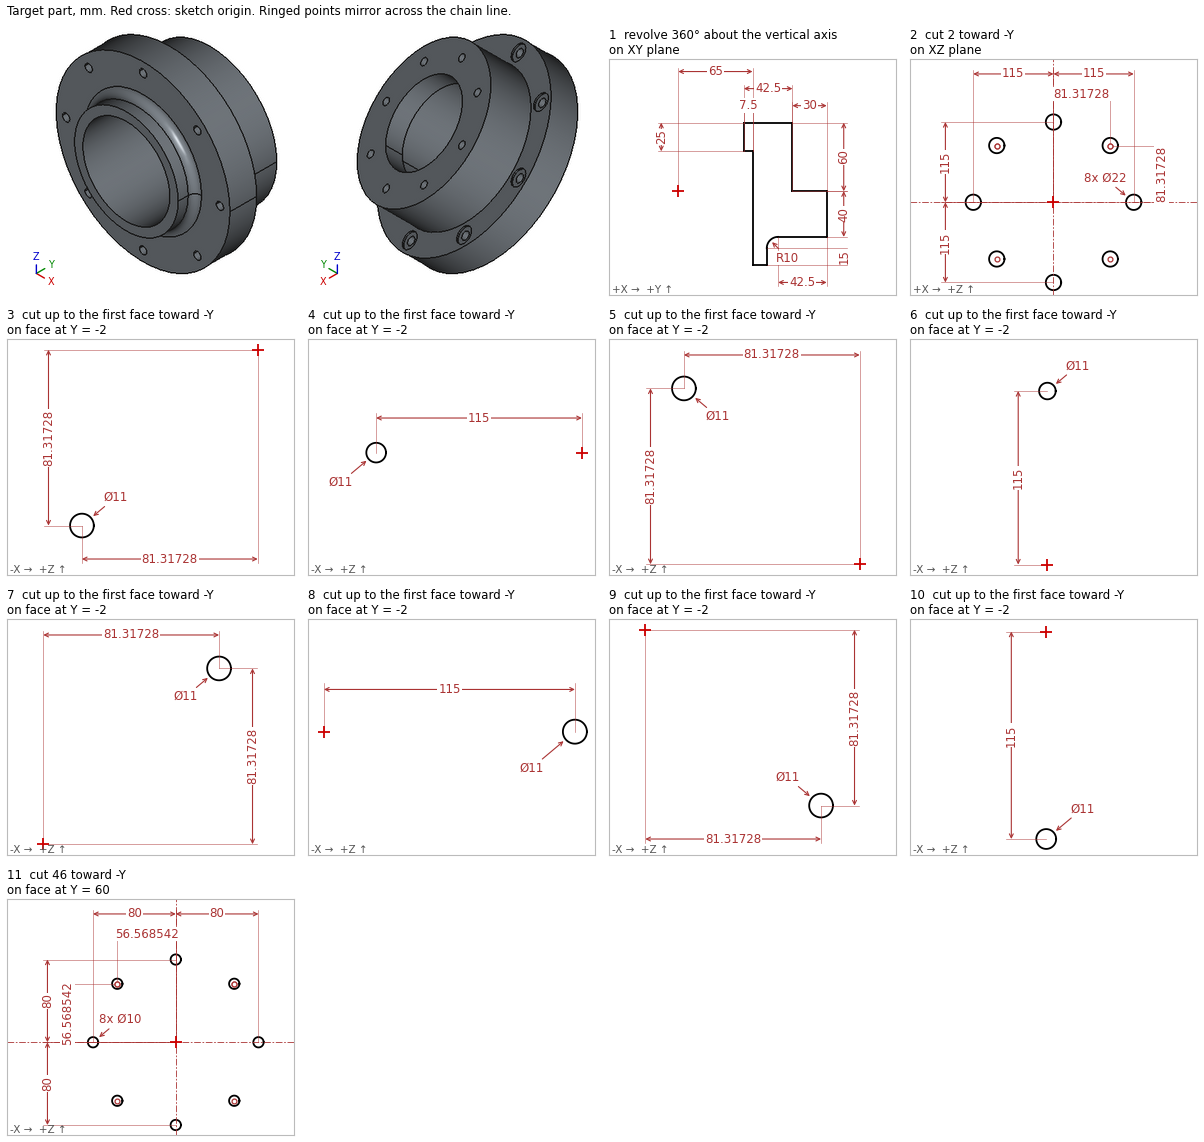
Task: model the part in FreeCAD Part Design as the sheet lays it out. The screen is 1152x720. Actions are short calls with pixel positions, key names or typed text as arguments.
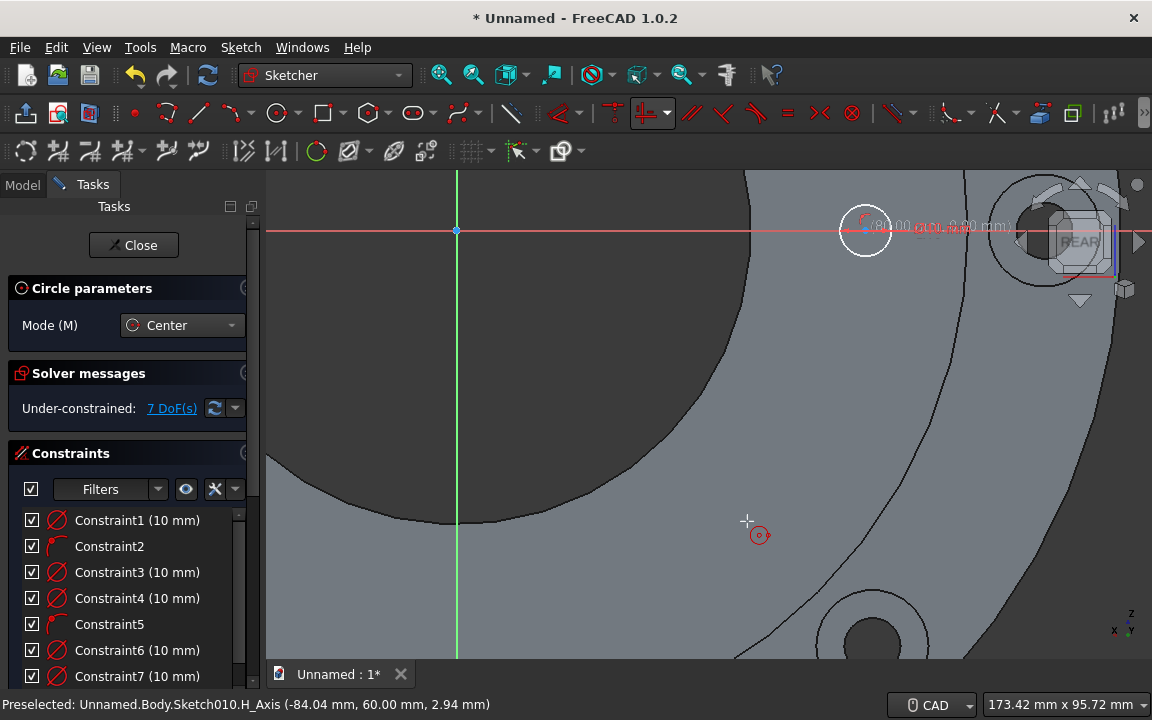
click(746, 520)
move(764, 502)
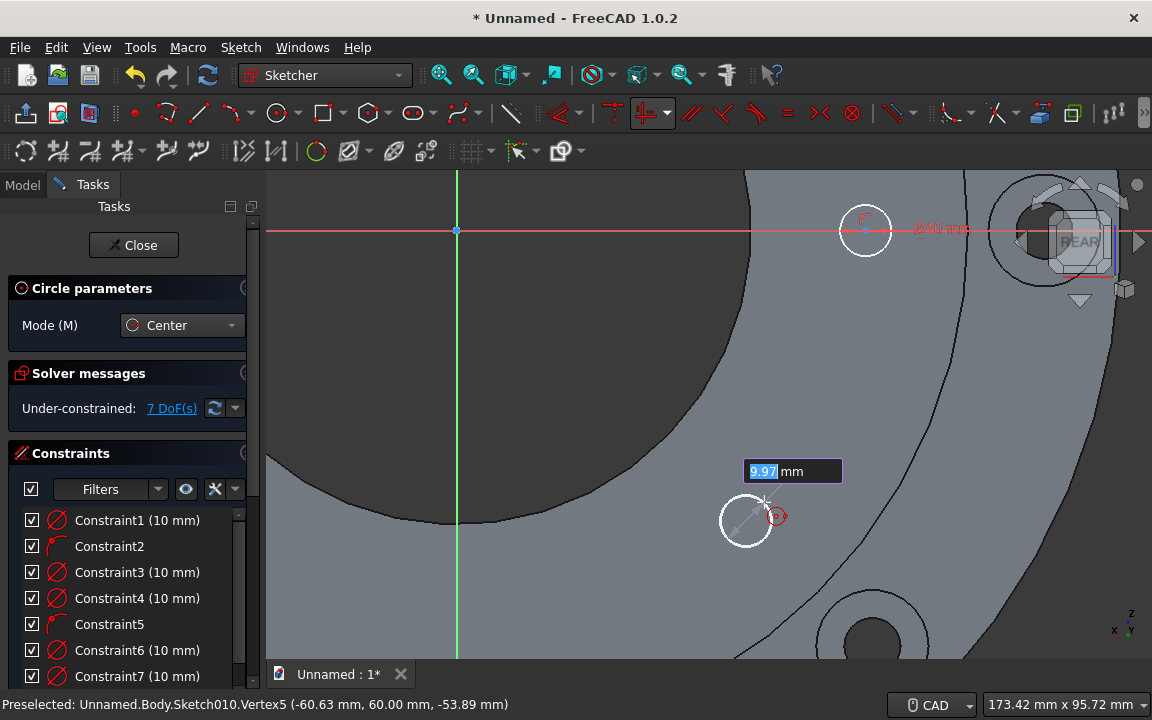
text(10)
key(Return)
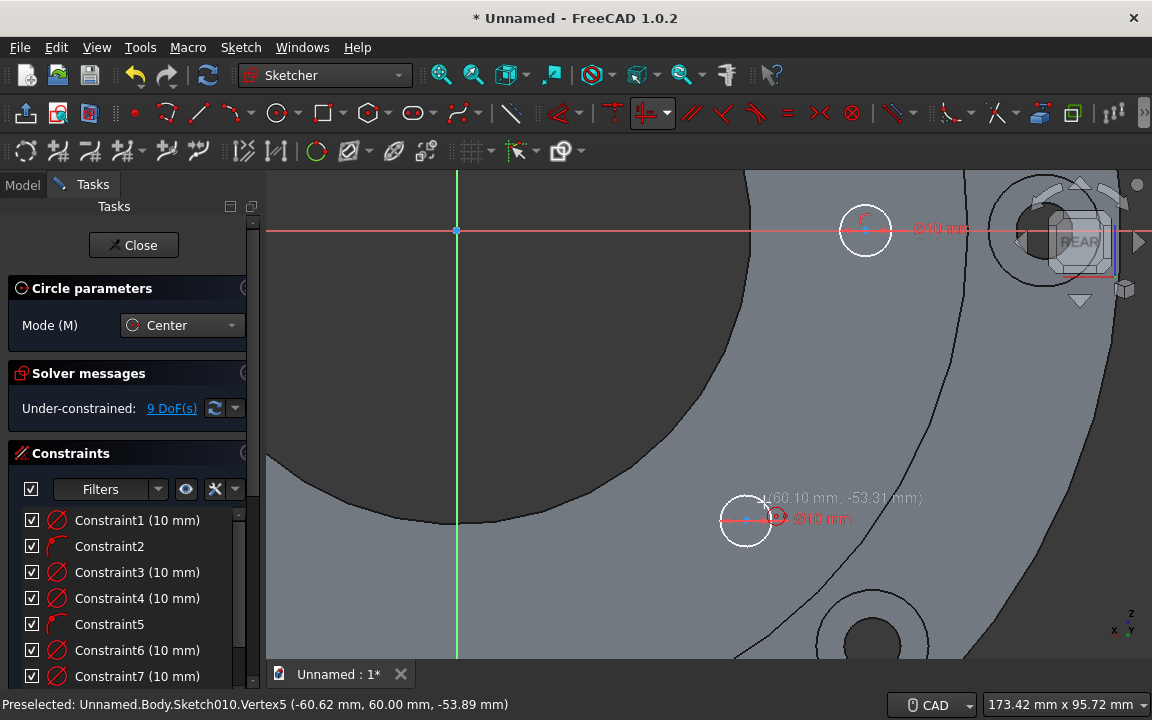
scroll(747, 521, down, 5)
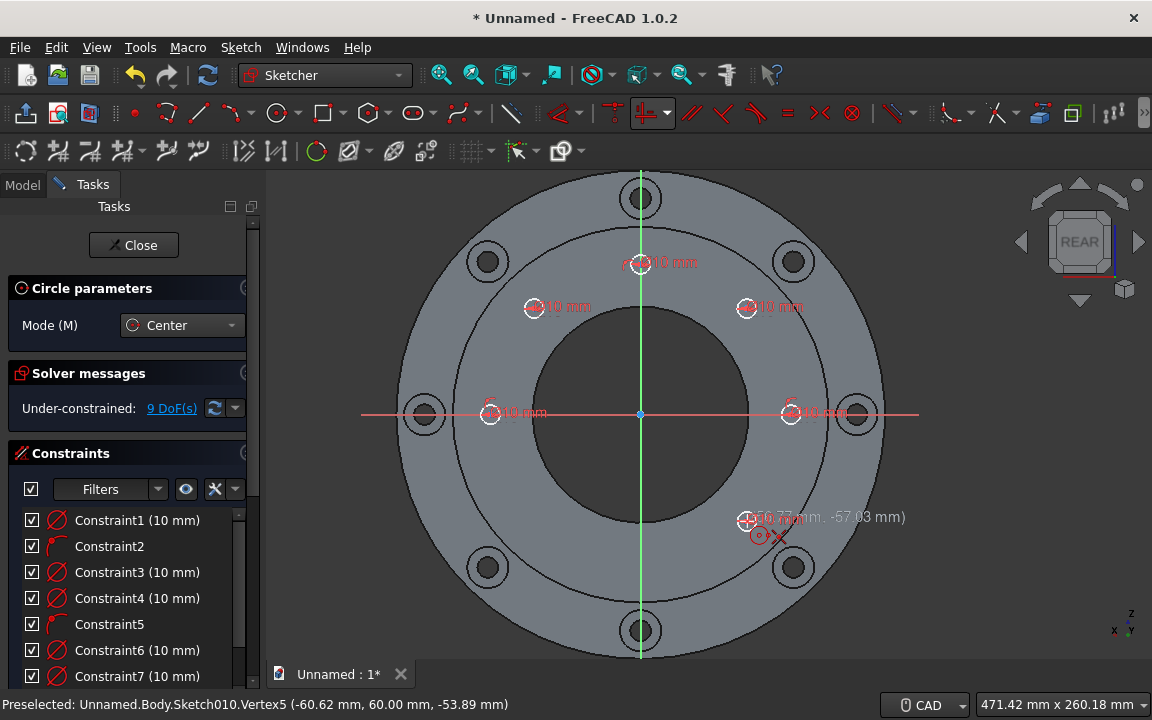
scroll(641, 565, up, 5)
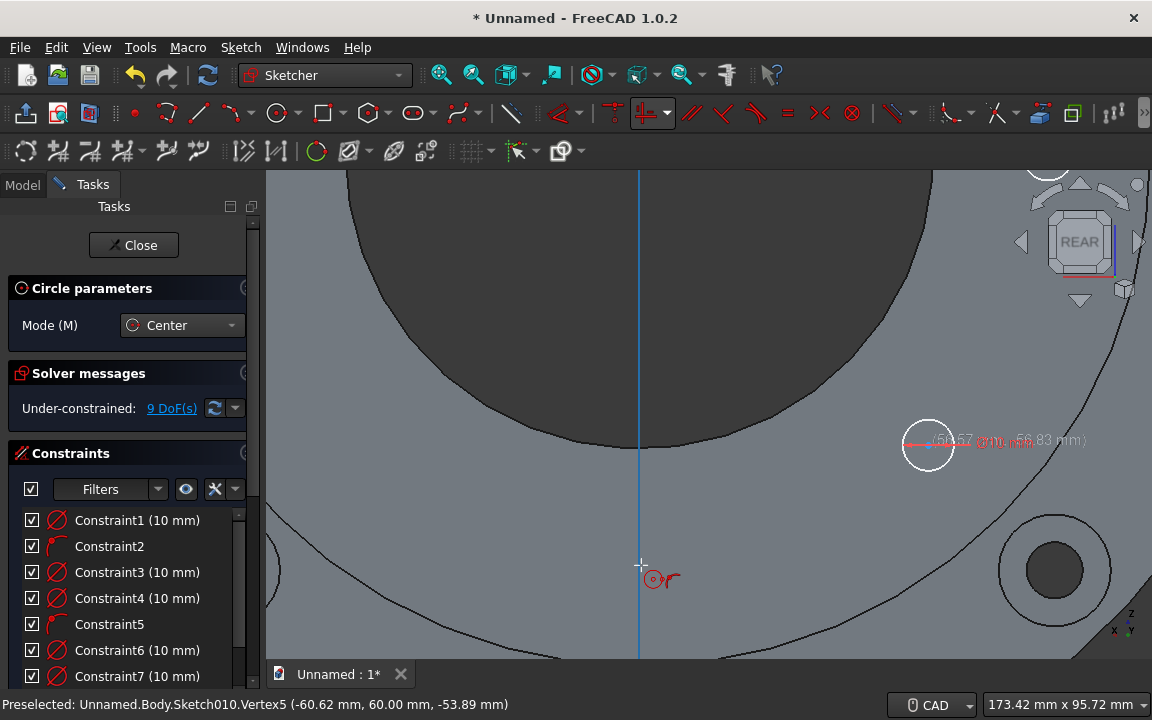
click(639, 564)
move(657, 546)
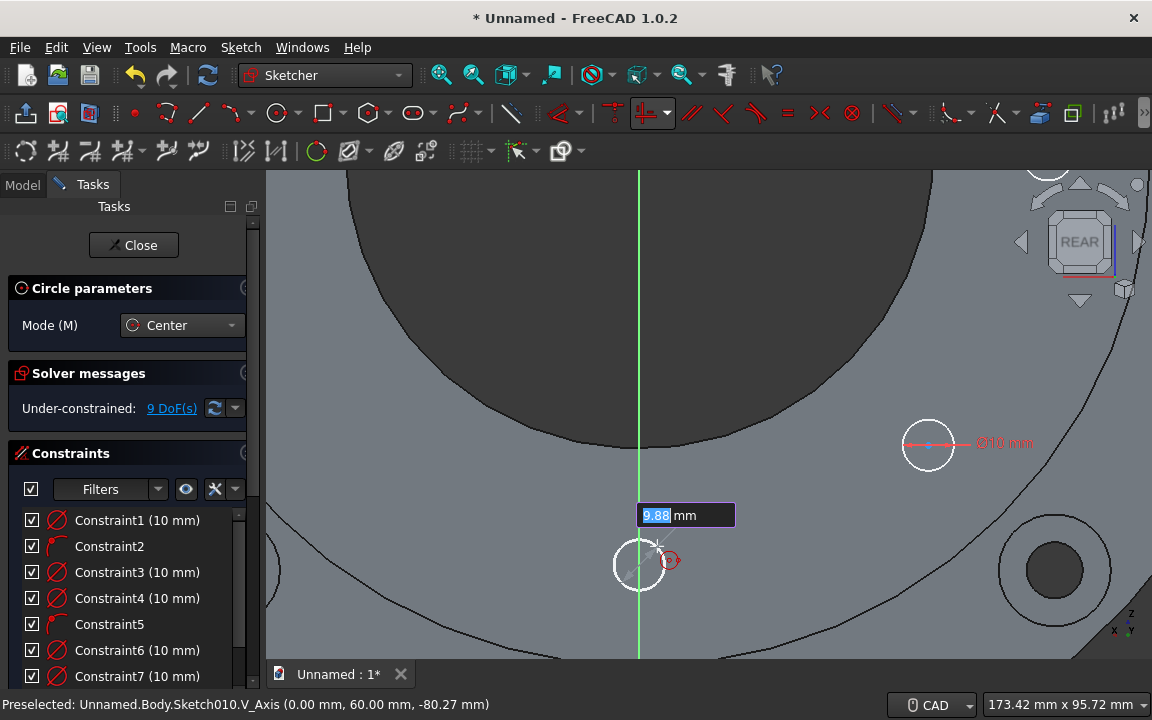
text(10)
key(Return)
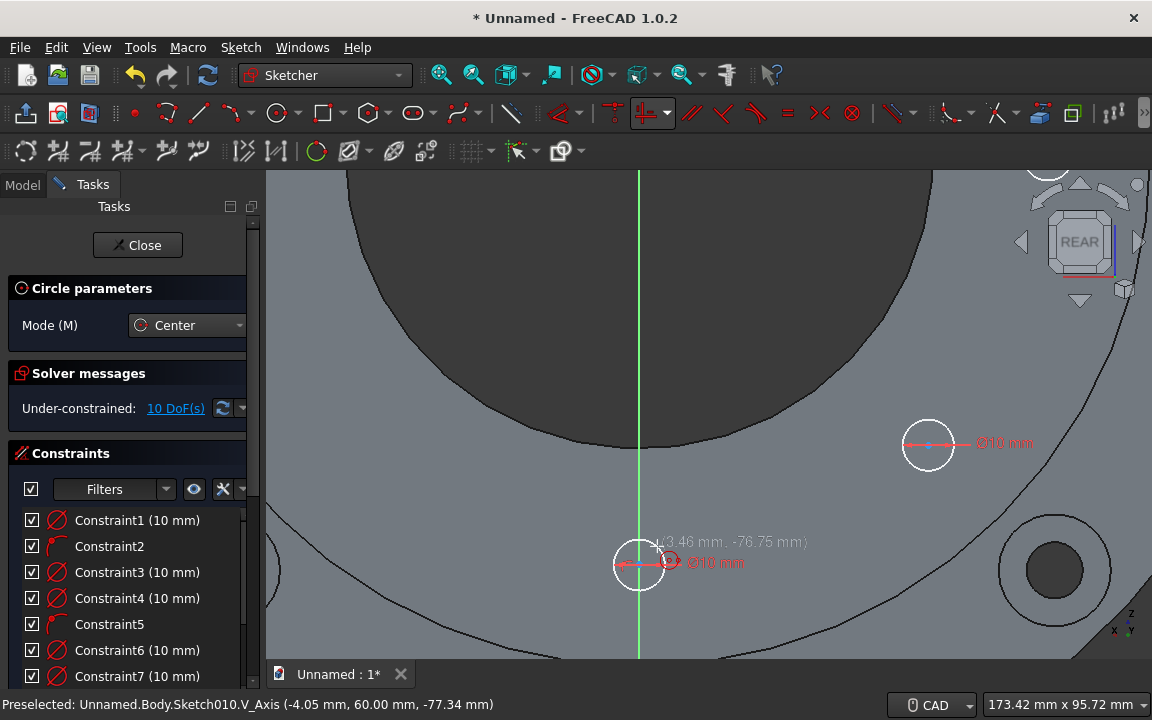
click(350, 444)
move(368, 426)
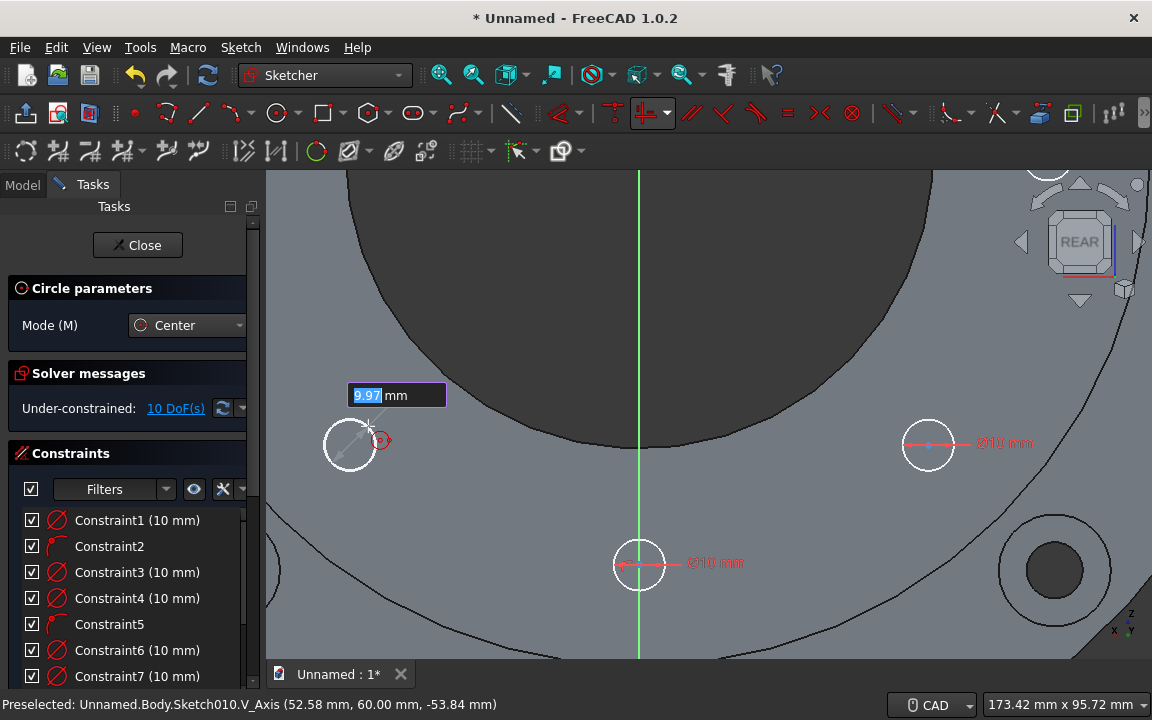
text(10)
key(Return)
key(Escape)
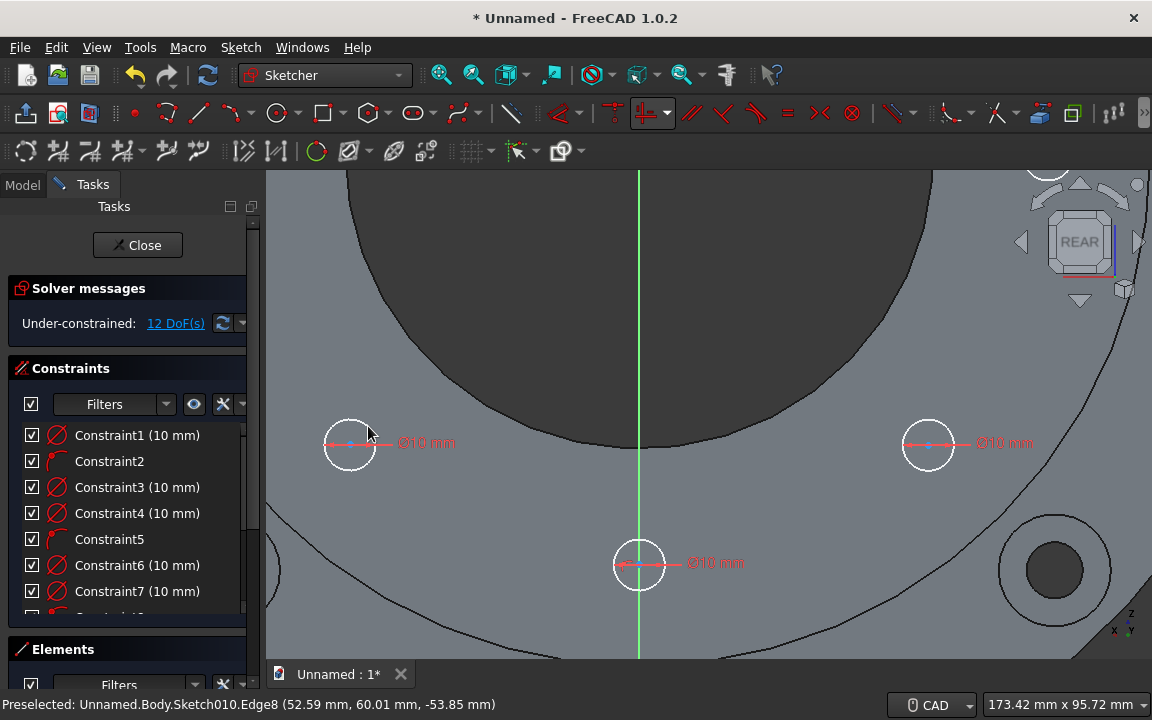
scroll(641, 566, down, 5)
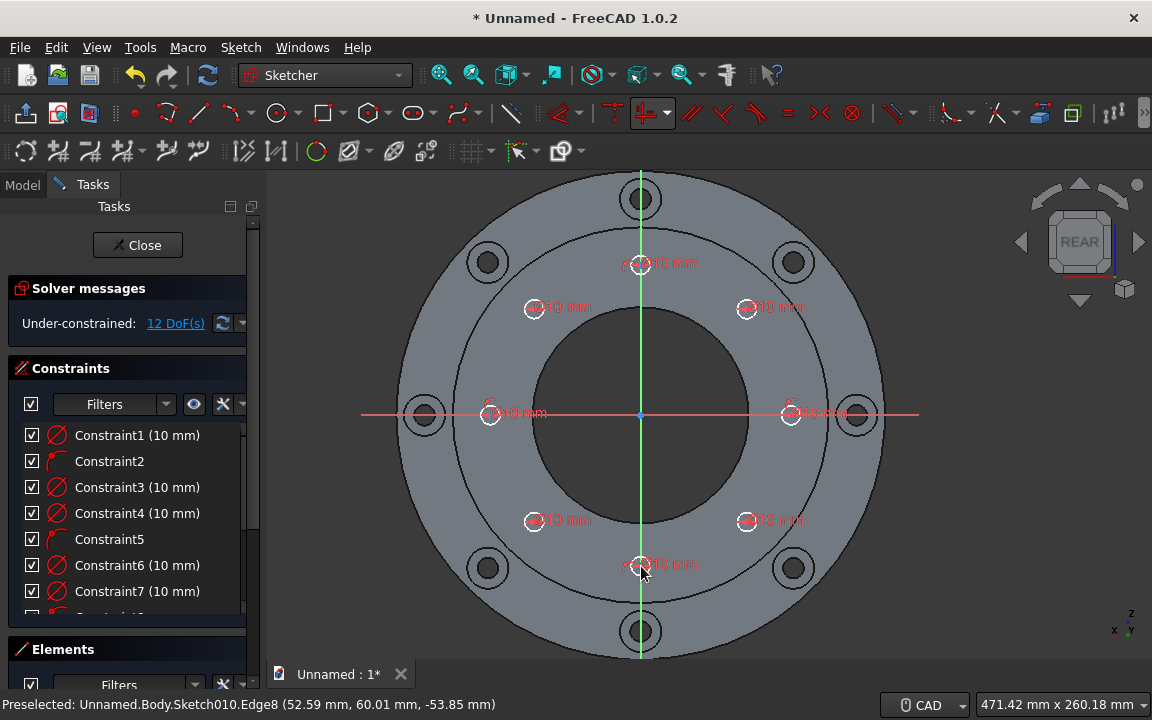
click(534, 309)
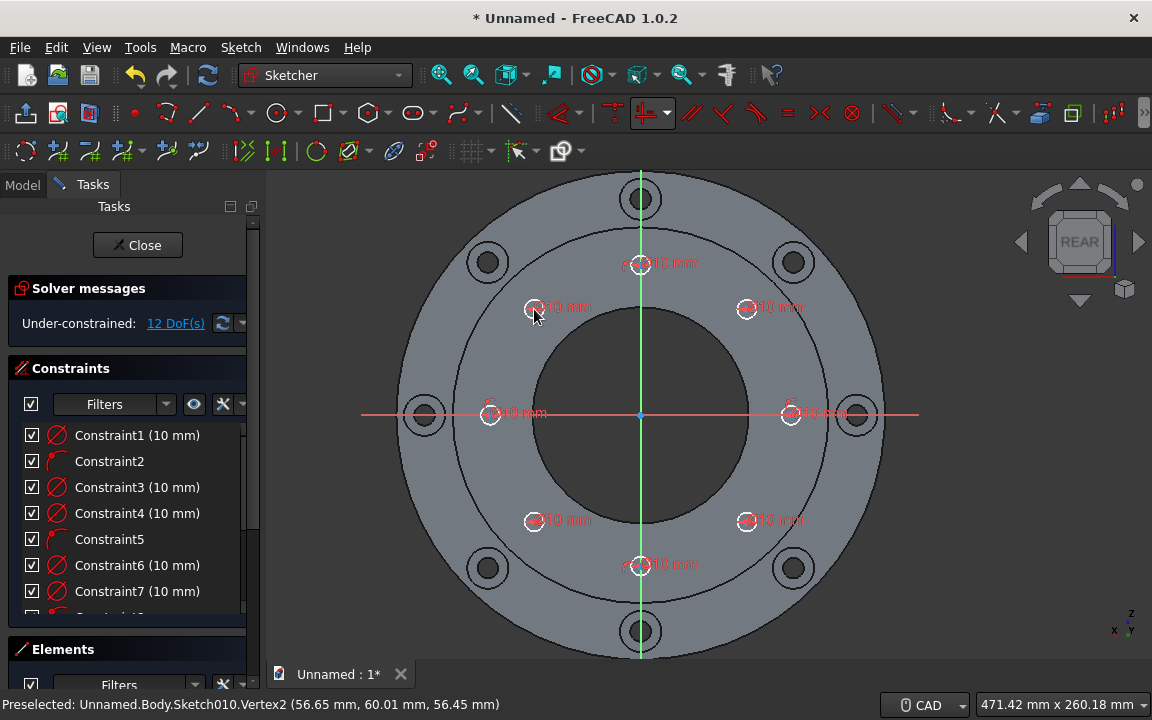
click(747, 309)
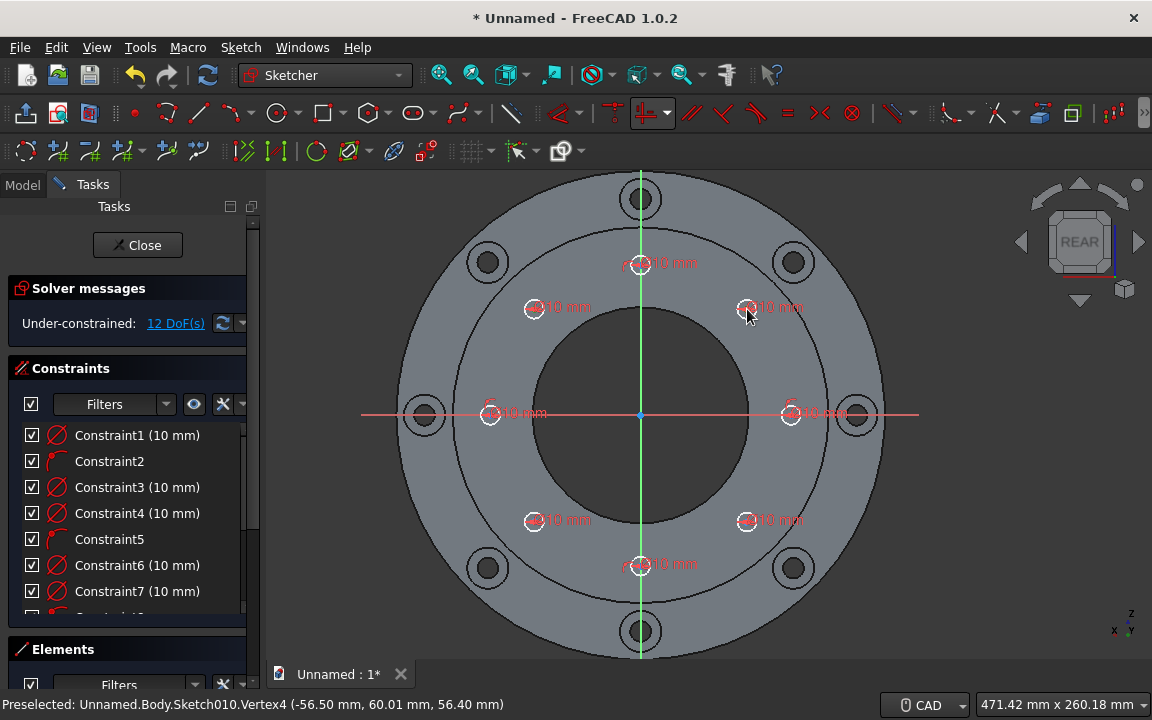
click(641, 507)